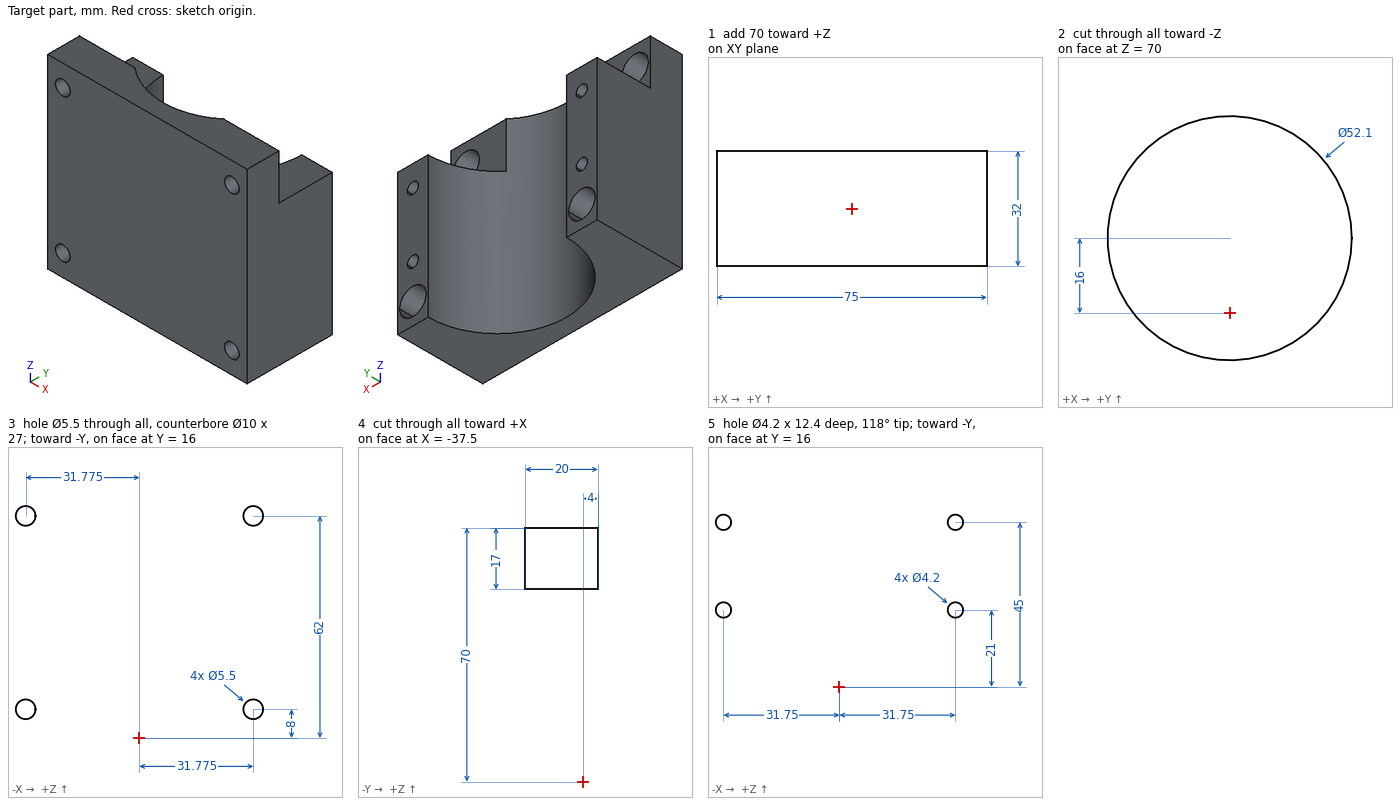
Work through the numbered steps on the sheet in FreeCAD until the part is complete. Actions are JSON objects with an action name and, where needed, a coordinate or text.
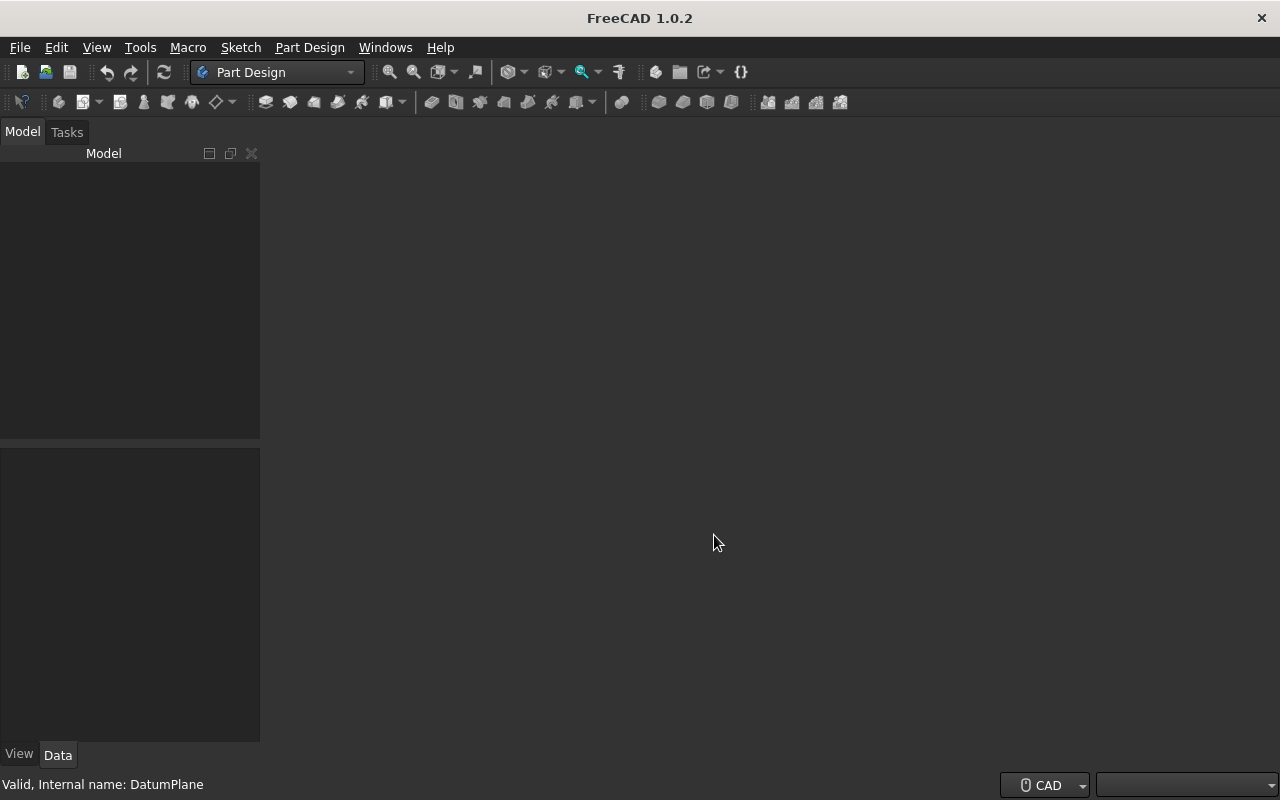
{"action": "left_click", "coordinate": [22, 72]}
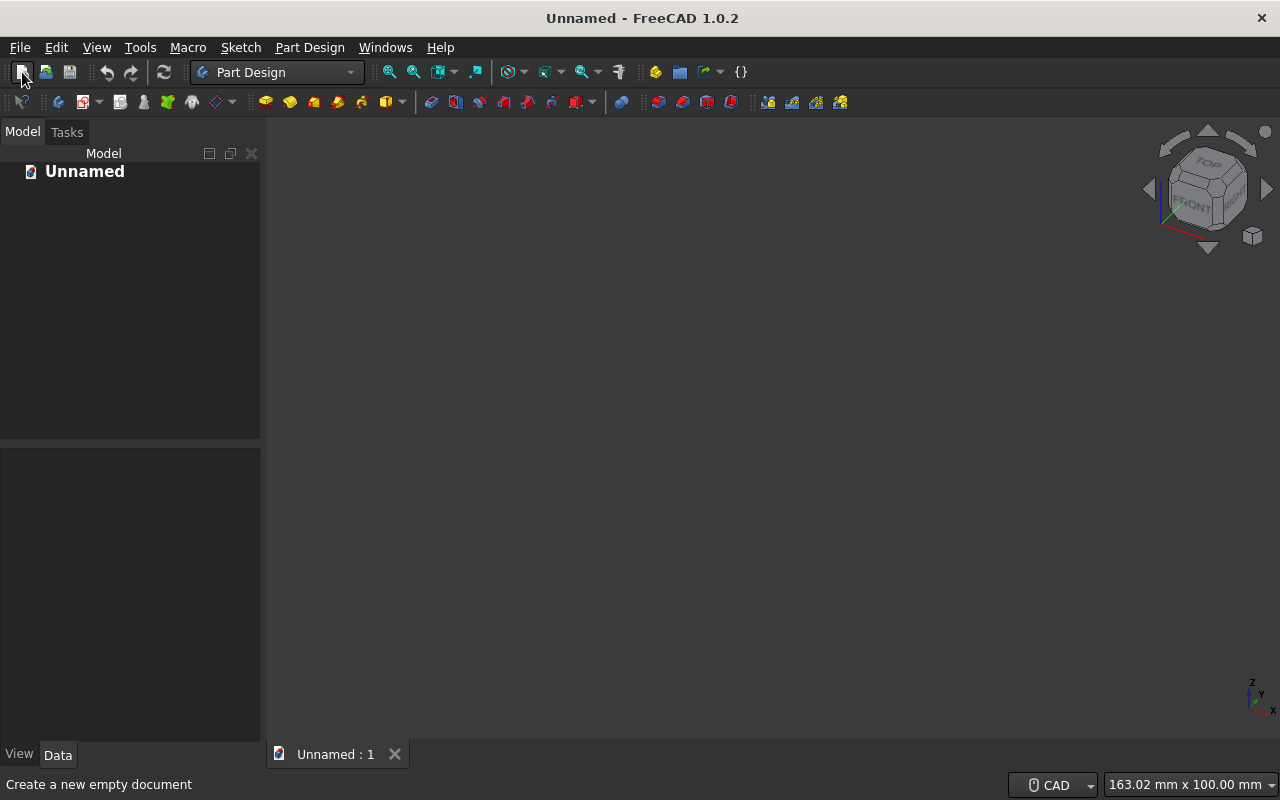
{"action": "left_click", "coordinate": [84, 102]}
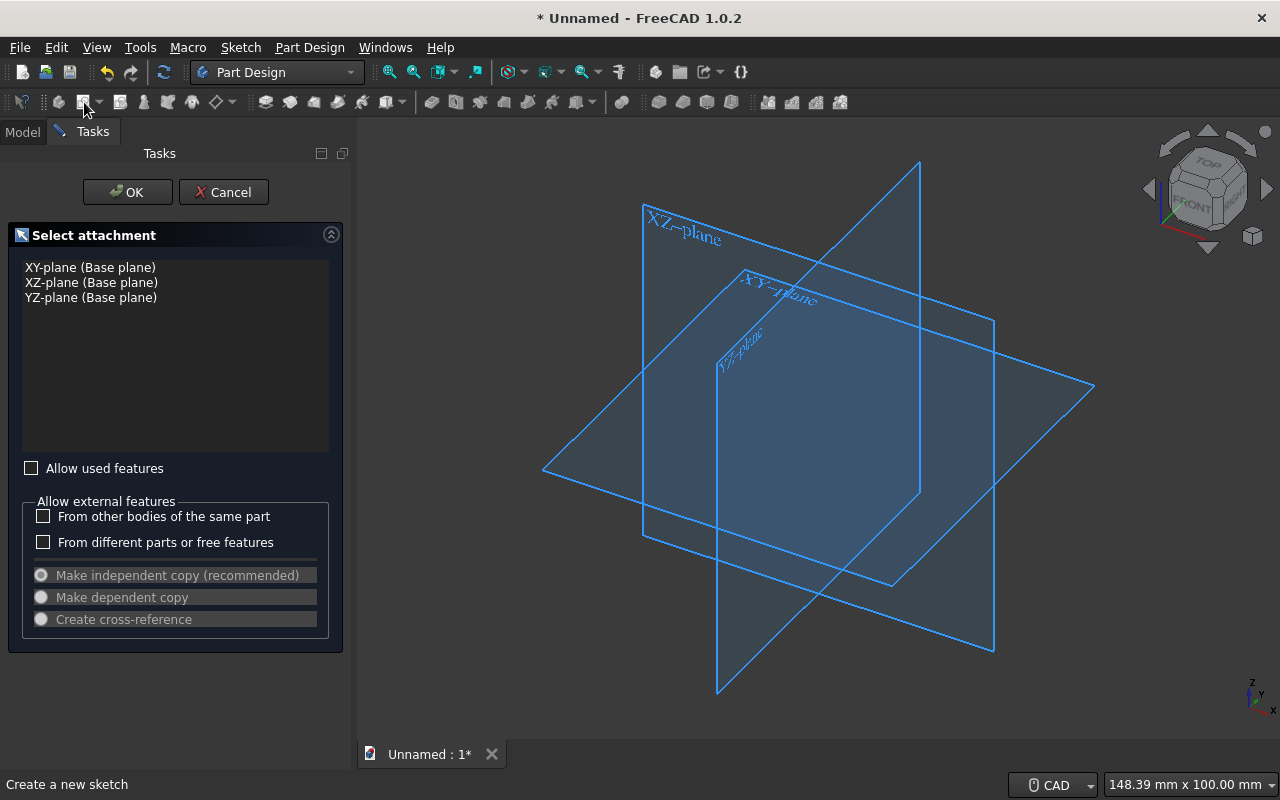
{"action": "left_click", "coordinate": [82, 268]}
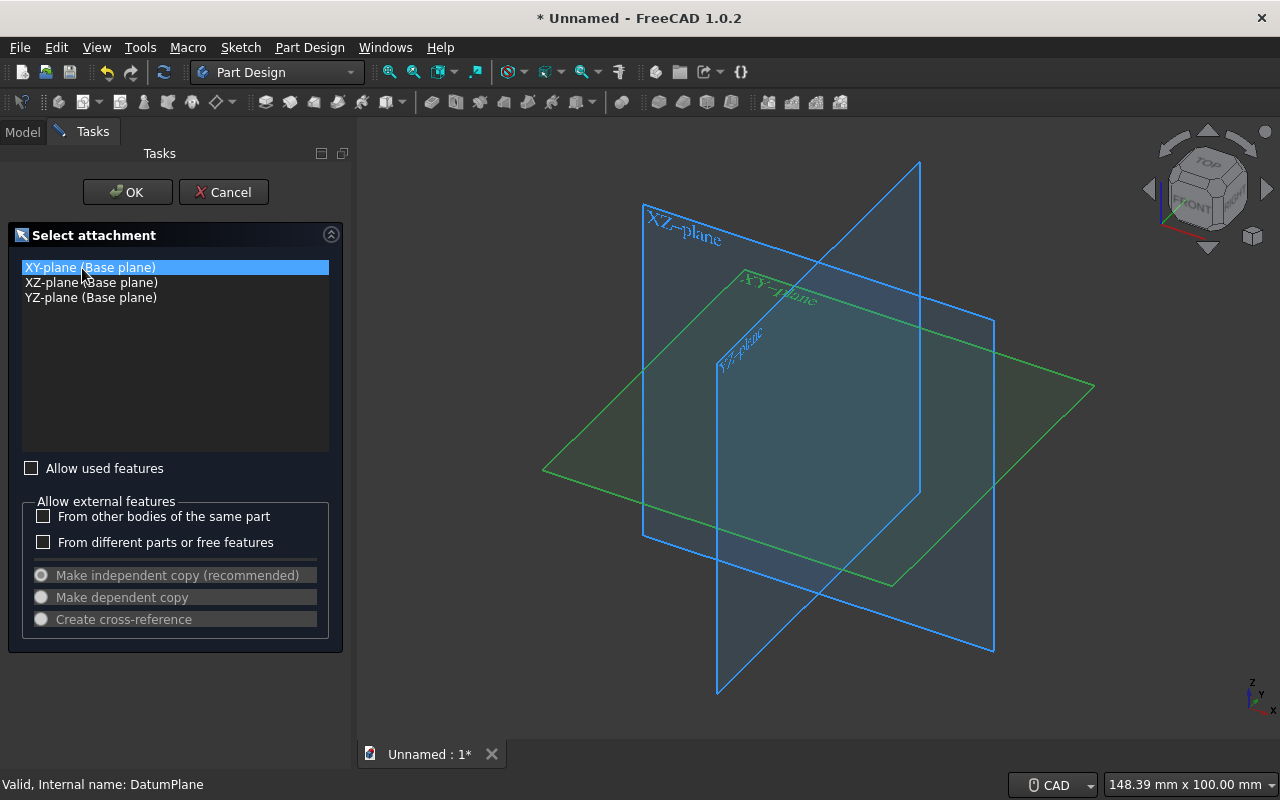
{"action": "left_click", "coordinate": [128, 192]}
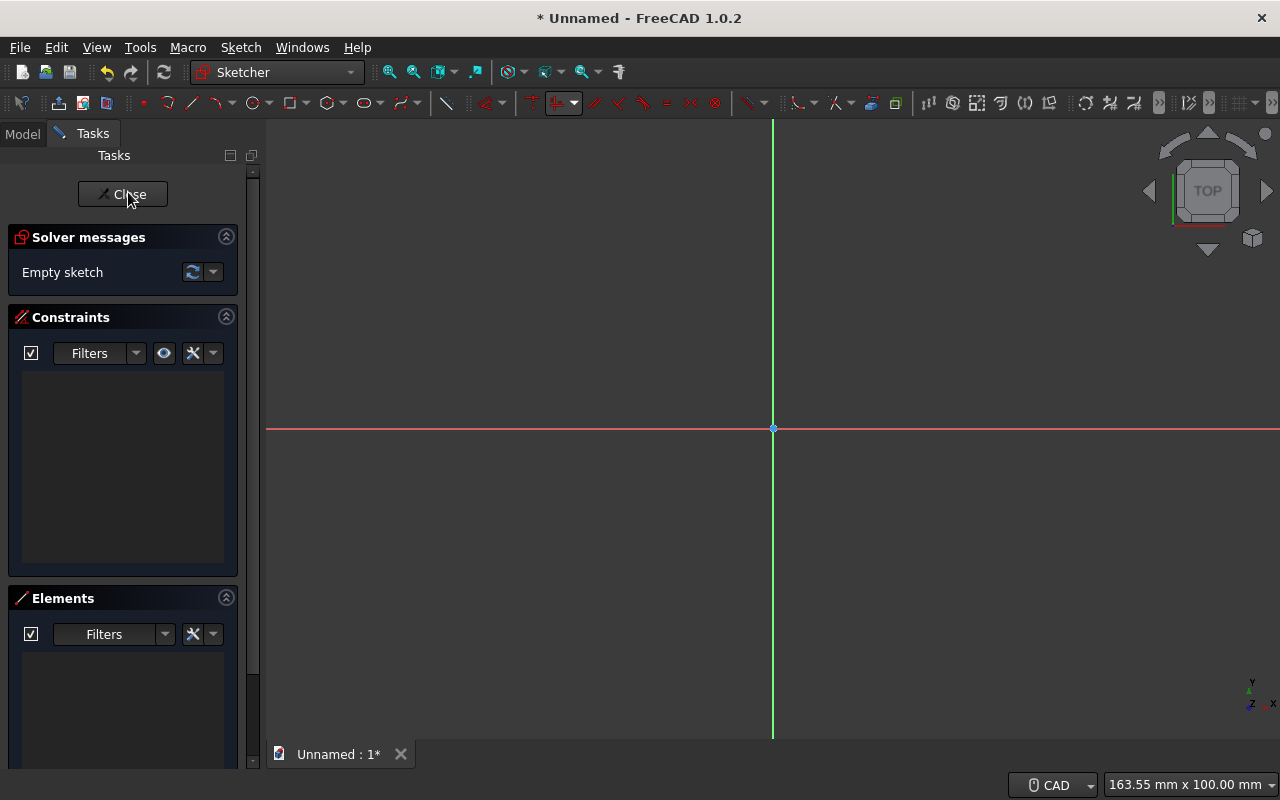
{"action": "key", "text": "g v"}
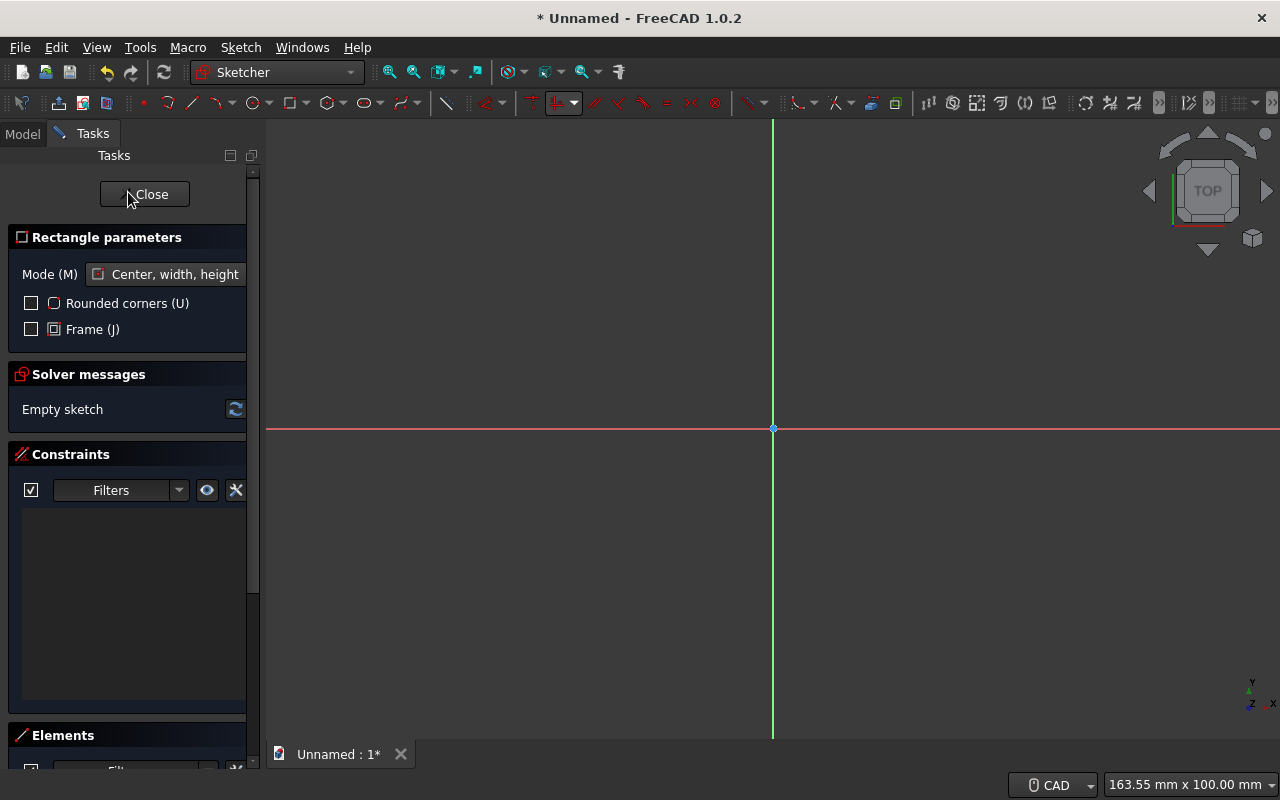
{"action": "left_click", "coordinate": [773, 429]}
{"action": "left_click", "coordinate": [1006, 330]}
{"action": "key", "text": "Escape"}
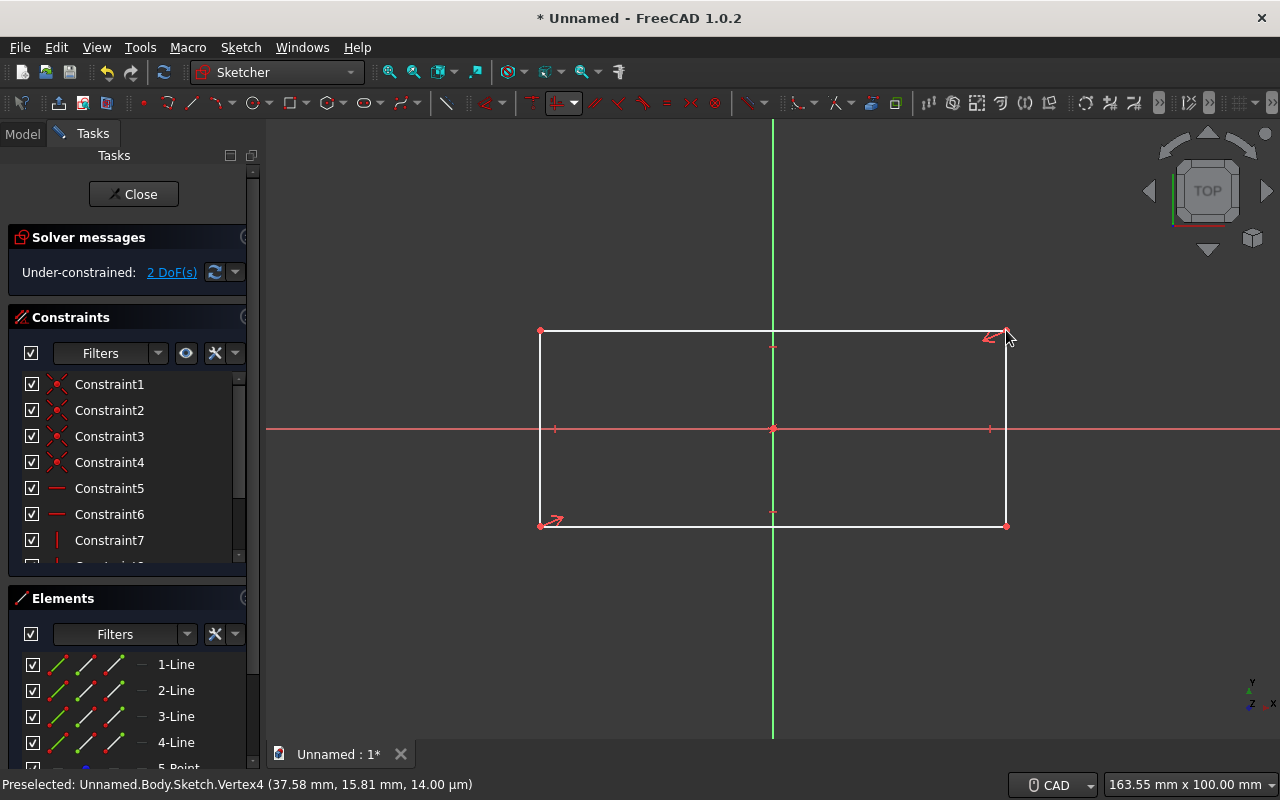
{"action": "left_click", "coordinate": [486, 104]}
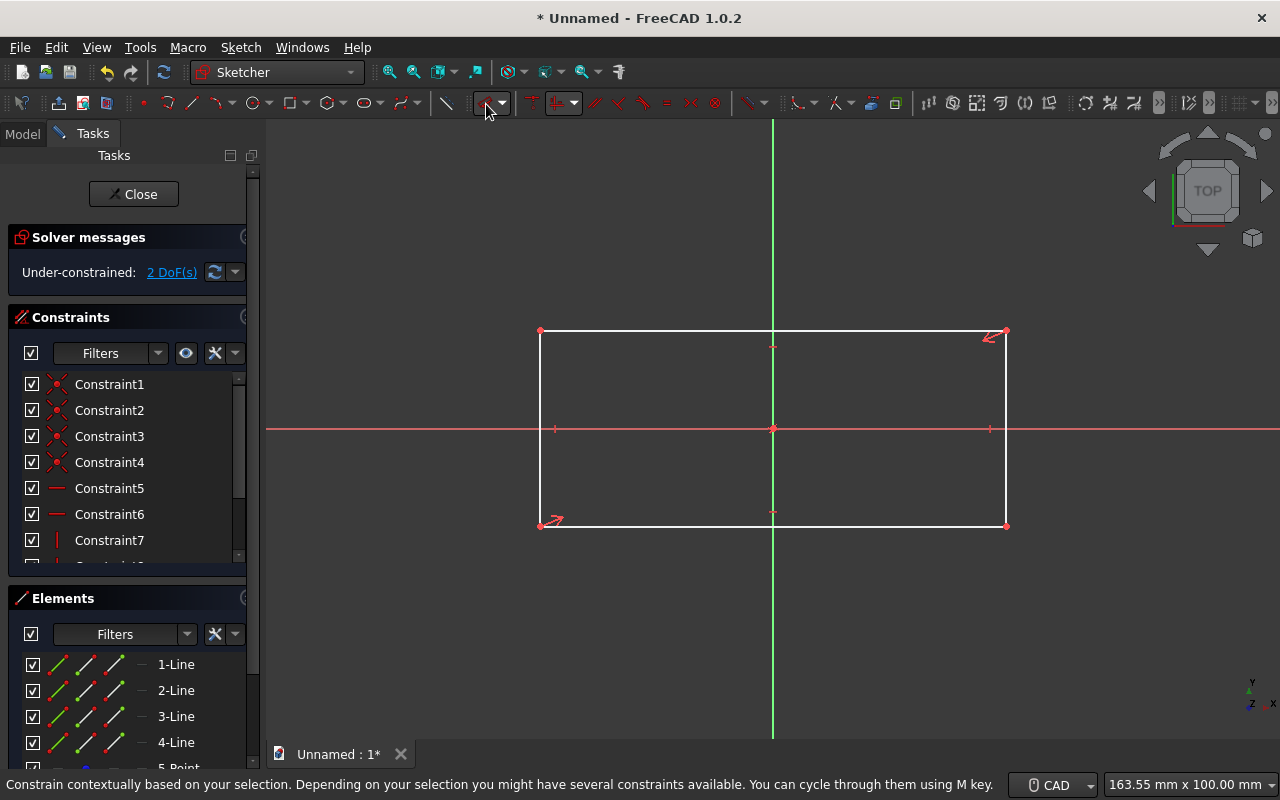
{"action": "left_click", "coordinate": [680, 527]}
{"action": "left_click", "coordinate": [666, 561]}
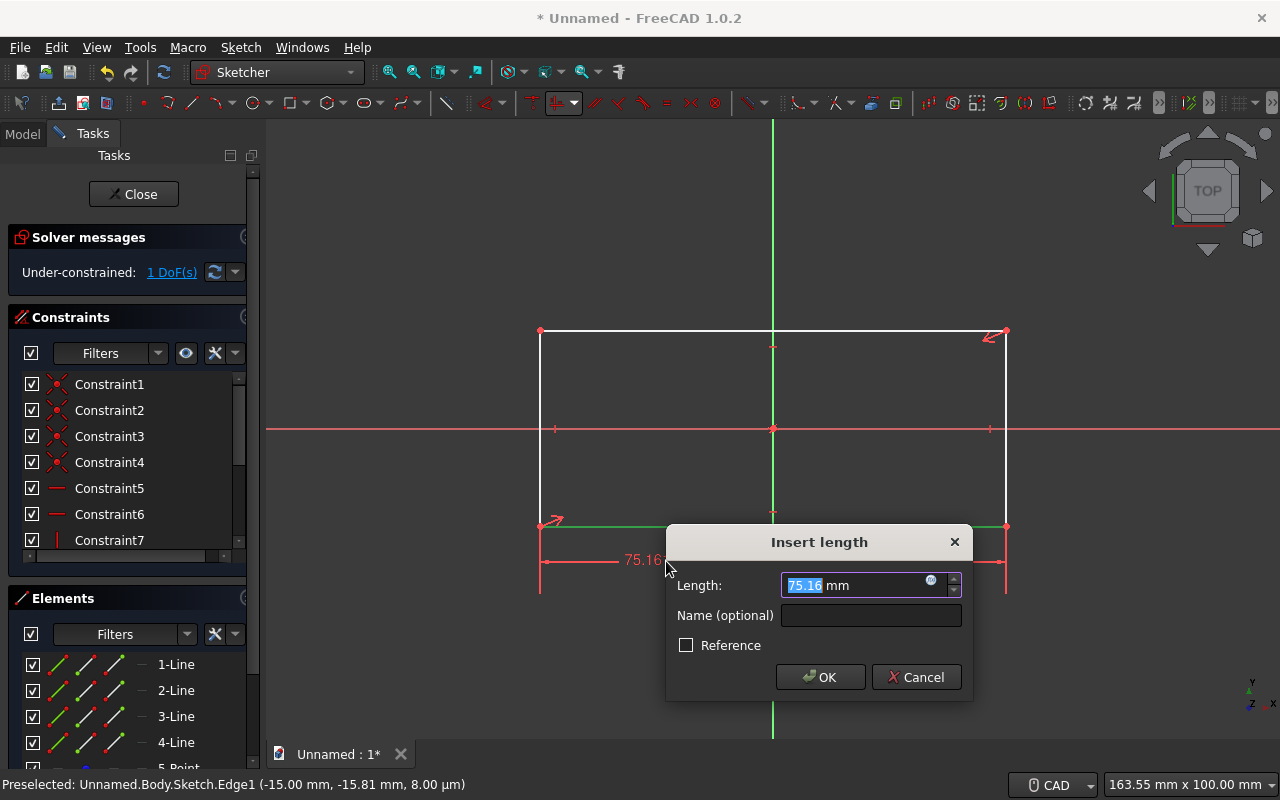
{"action": "type", "text": "75"}
{"action": "key", "text": "Return"}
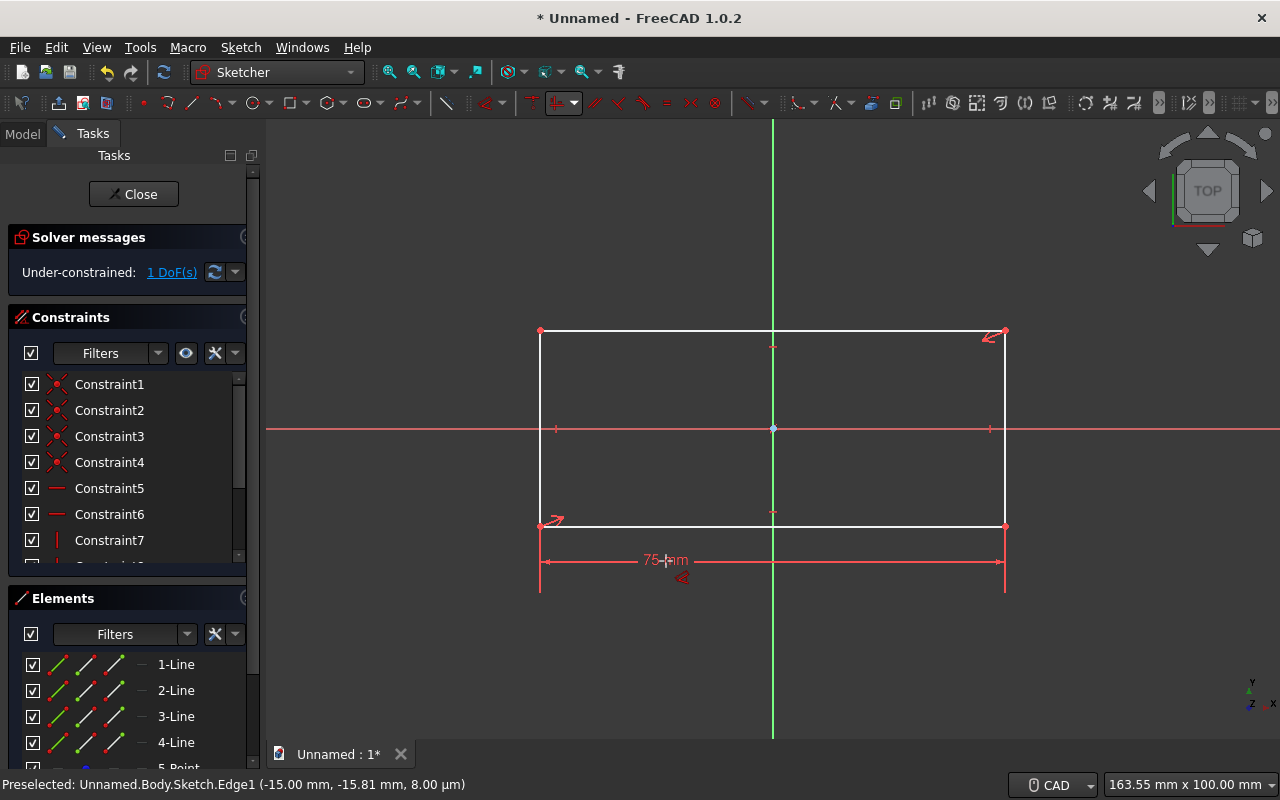
{"action": "left_click", "coordinate": [1006, 468]}
{"action": "left_click", "coordinate": [1040, 384]}